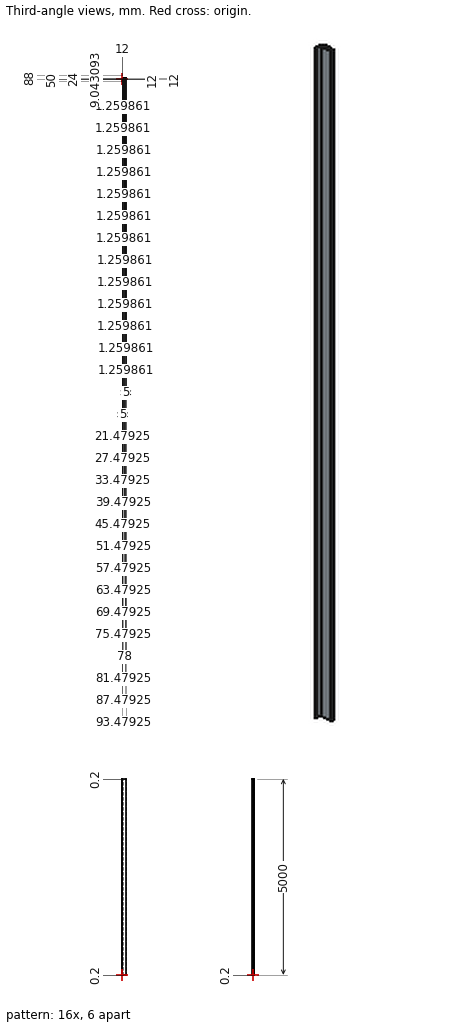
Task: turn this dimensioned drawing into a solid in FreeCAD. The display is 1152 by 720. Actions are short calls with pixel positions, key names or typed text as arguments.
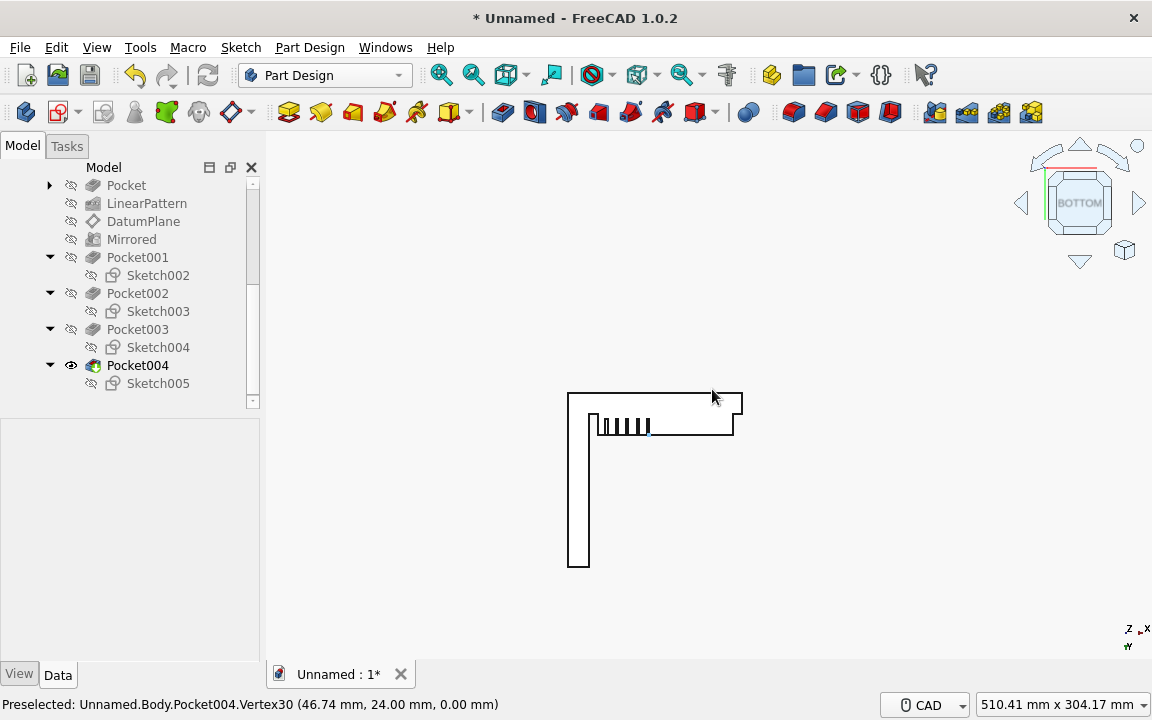
click(704, 405)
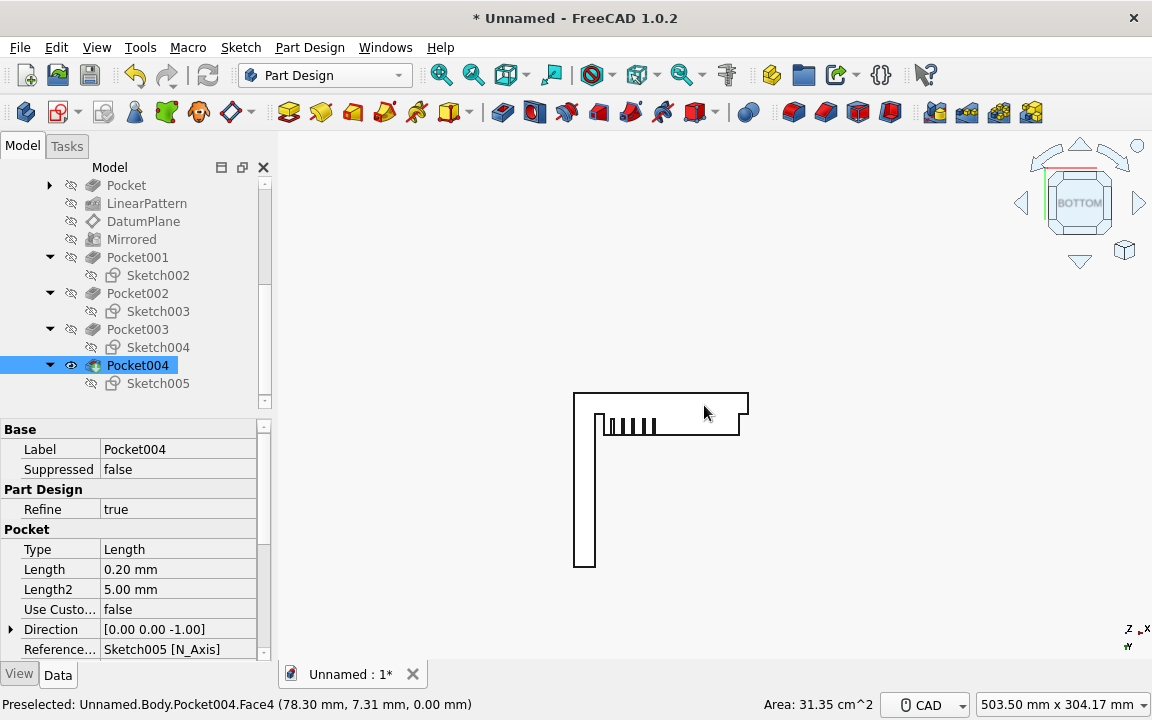
click(58, 112)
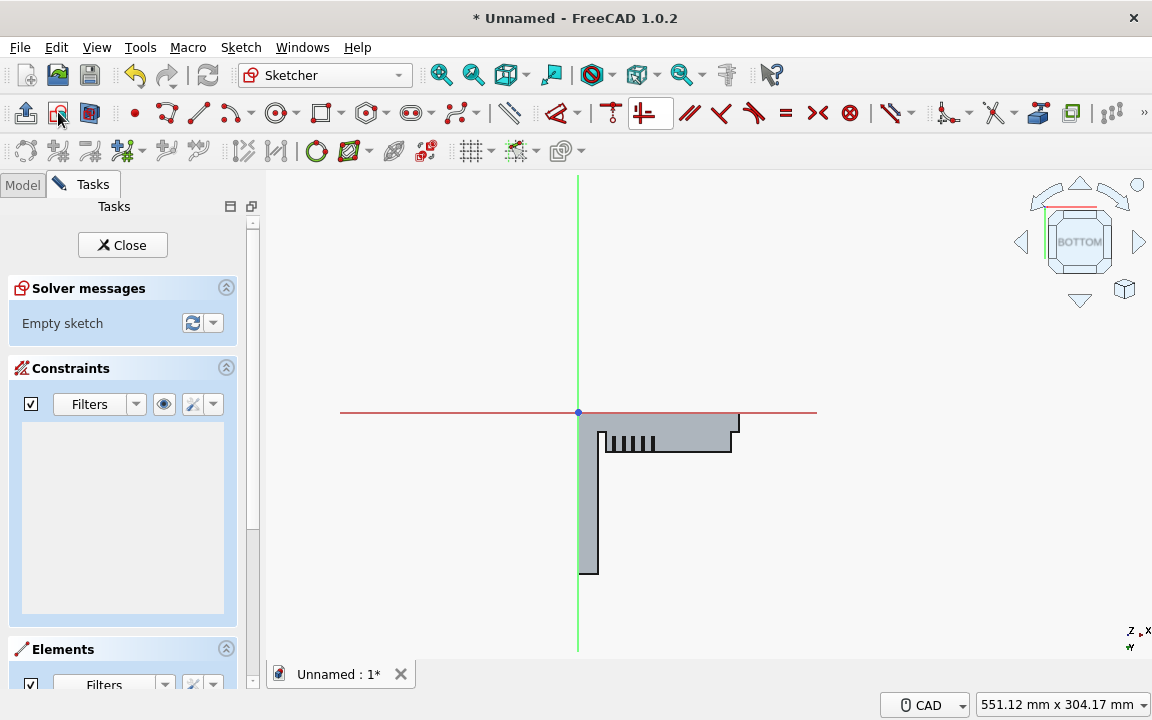
scroll(663, 446, up, 15)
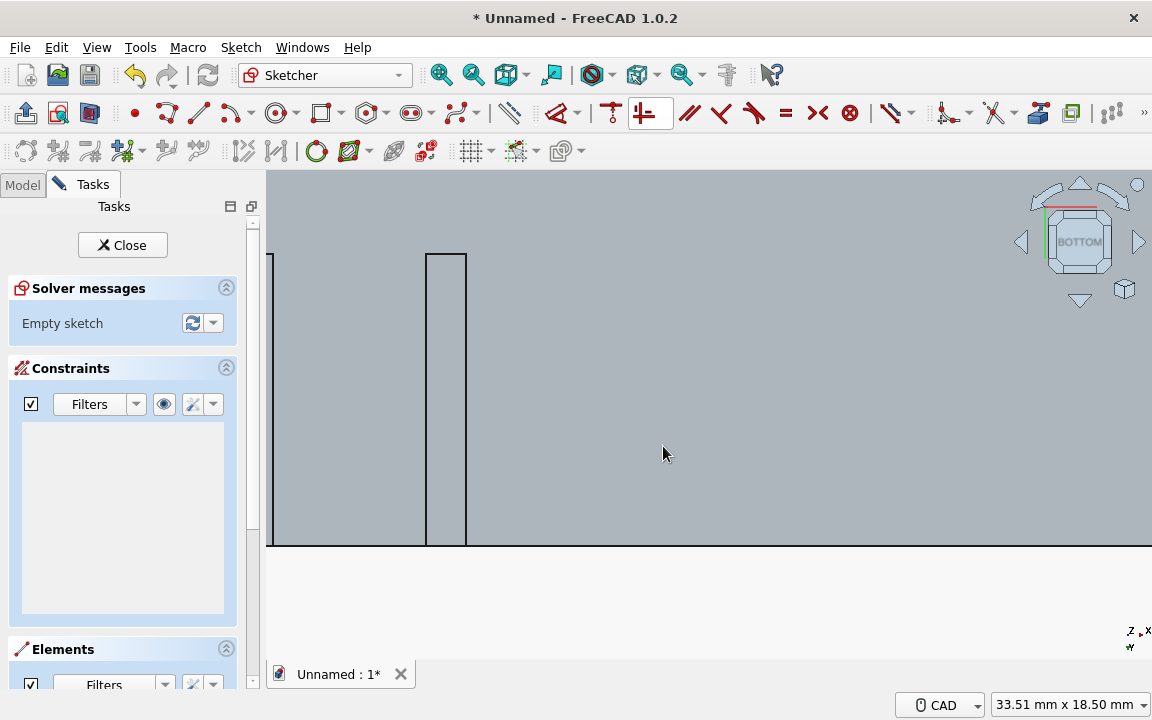
click(322, 114)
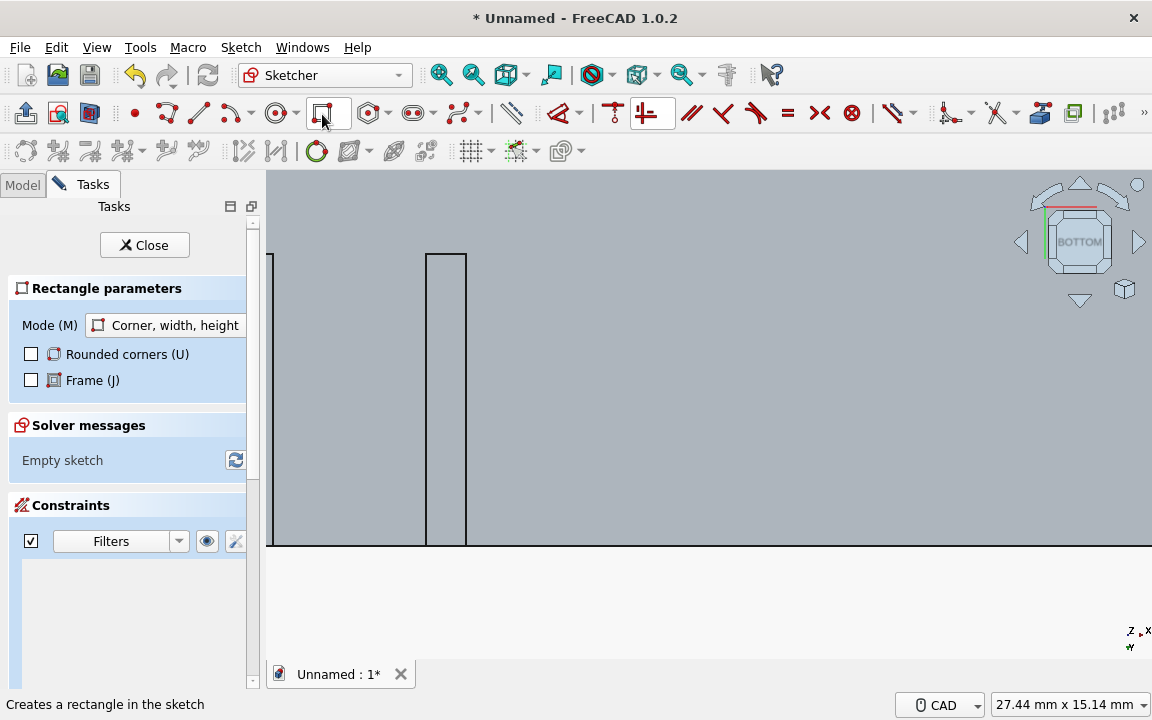
click(619, 254)
click(660, 546)
key(Escape)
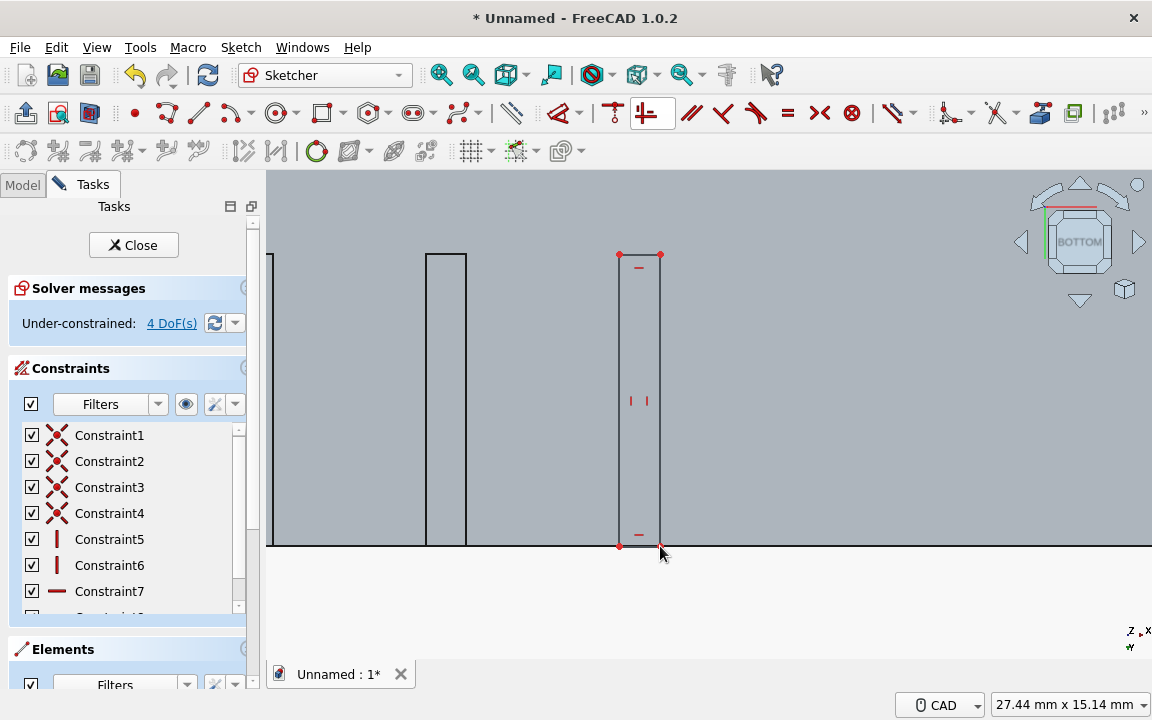
click(558, 114)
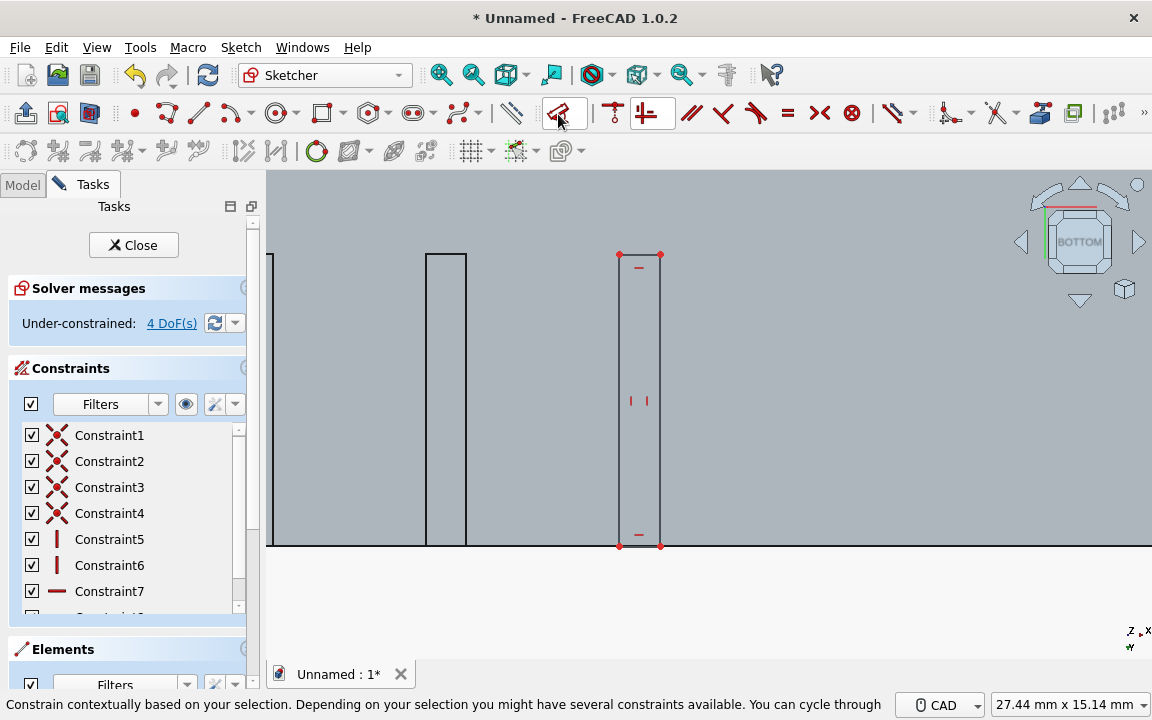
click(619, 547)
click(677, 373)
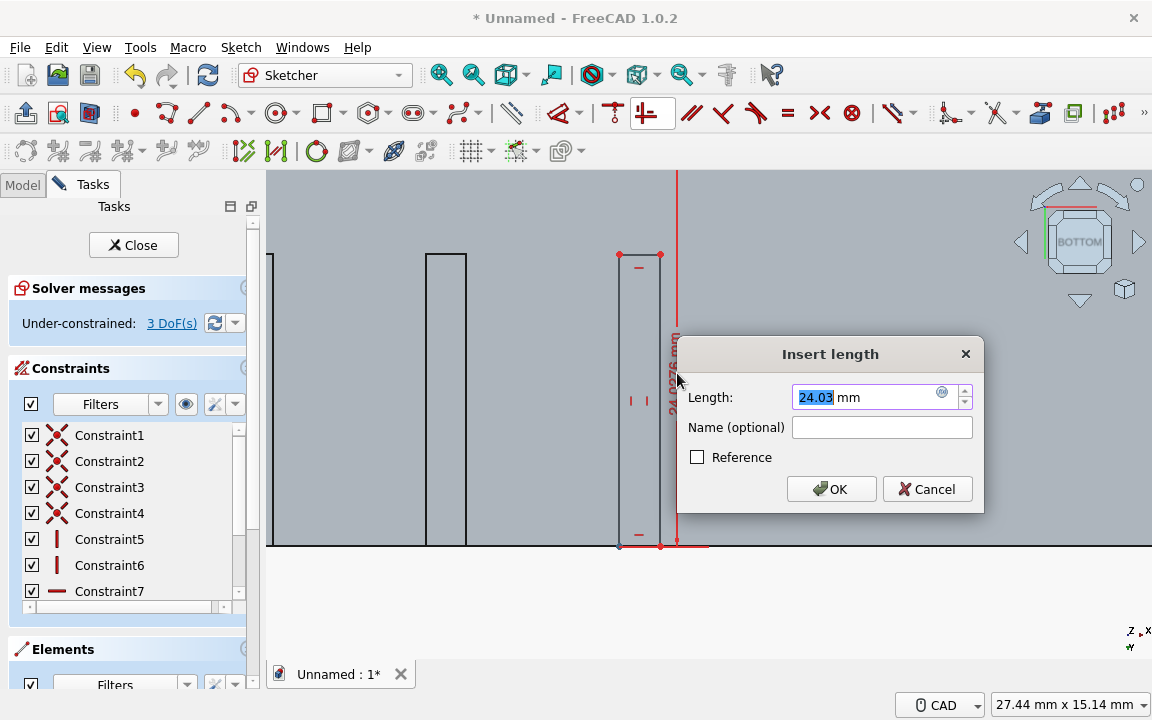
text(24)
key(Return)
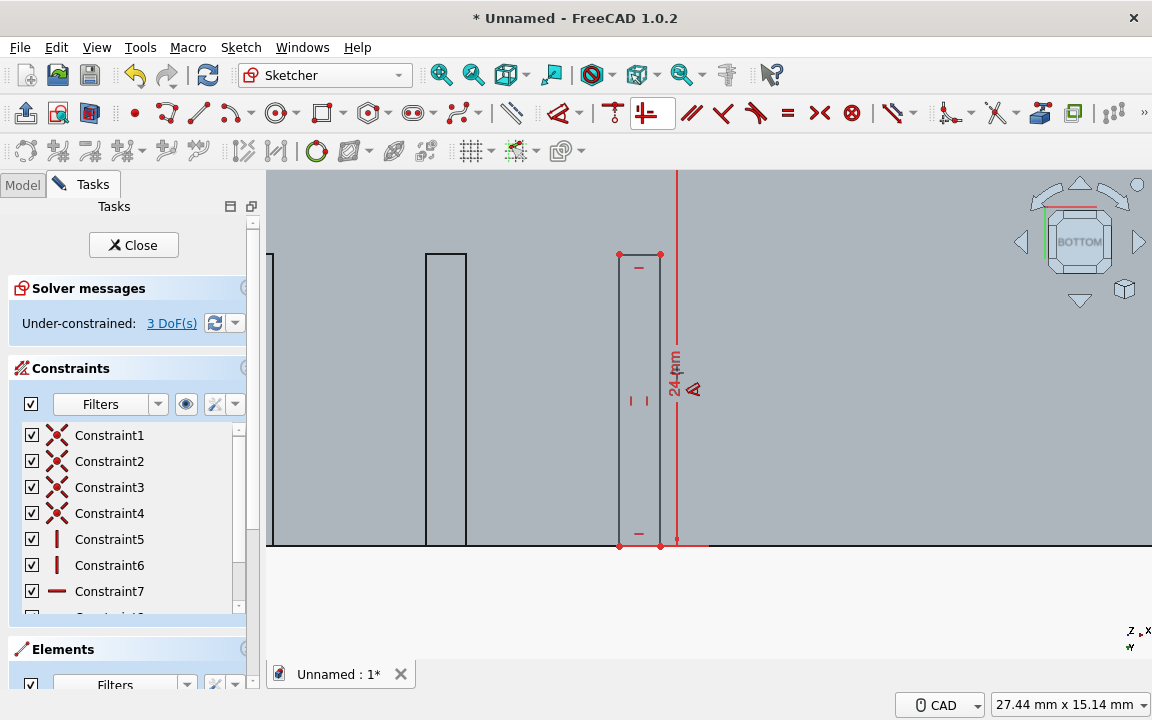
click(619, 342)
click(585, 401)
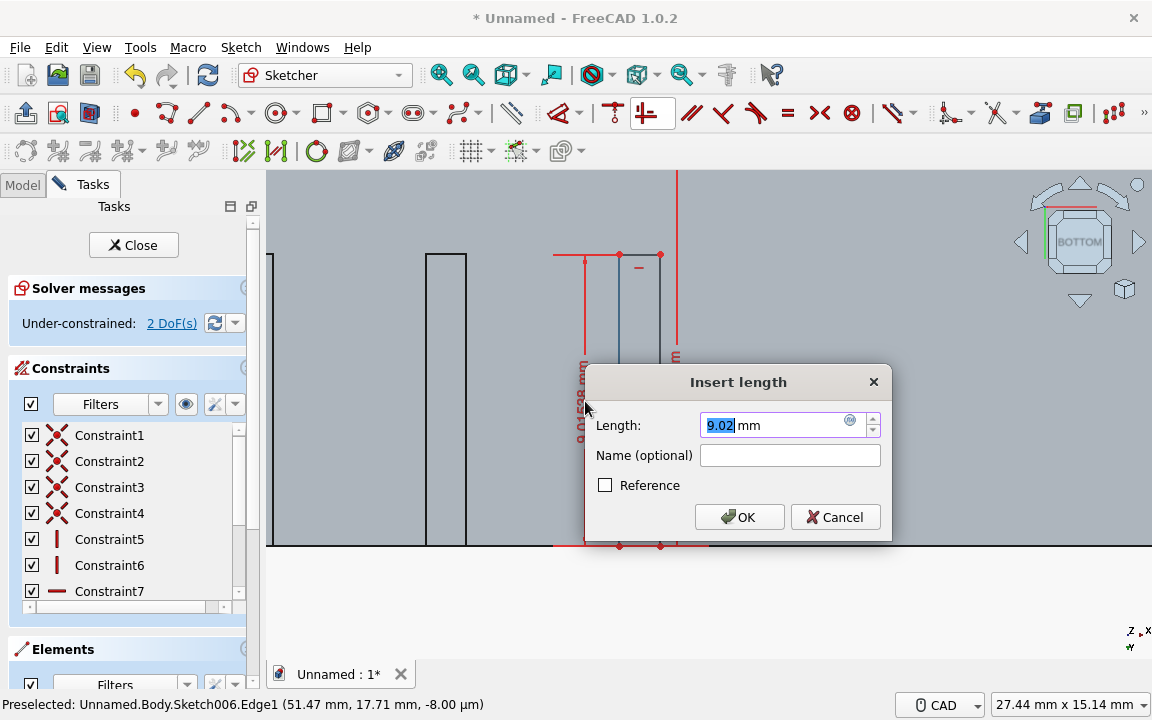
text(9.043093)
key(Return)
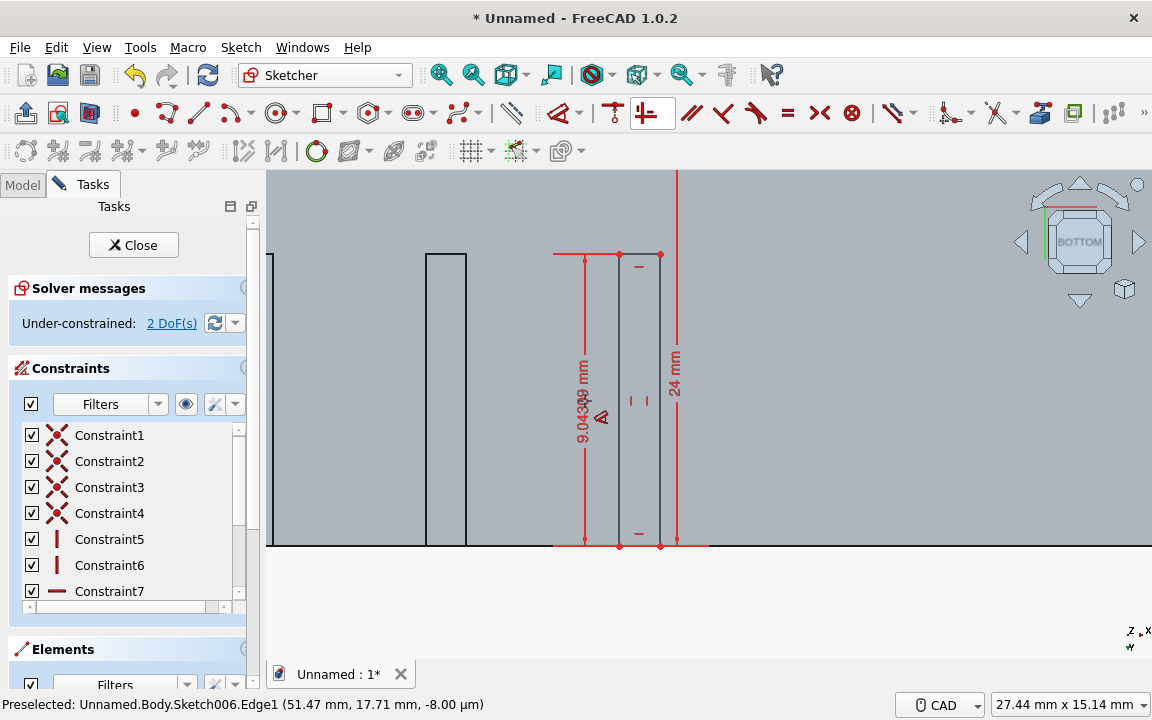
click(631, 546)
click(640, 580)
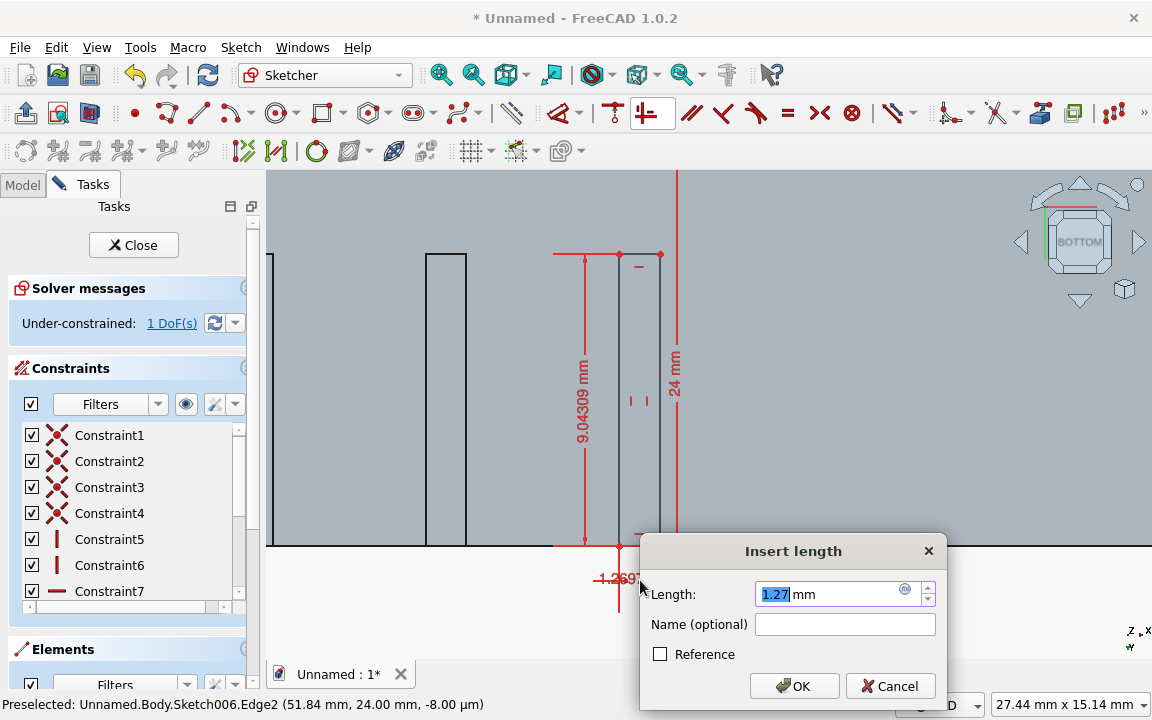
text(1.259861)
key(Return)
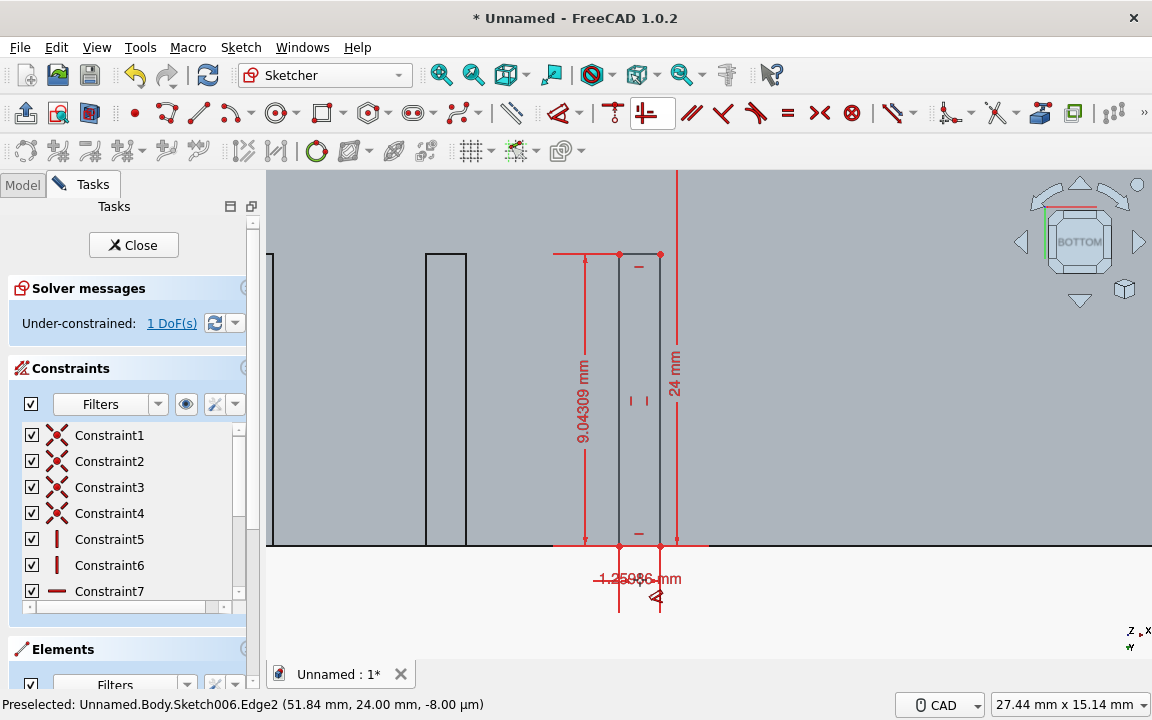
click(619, 254)
click(457, 288)